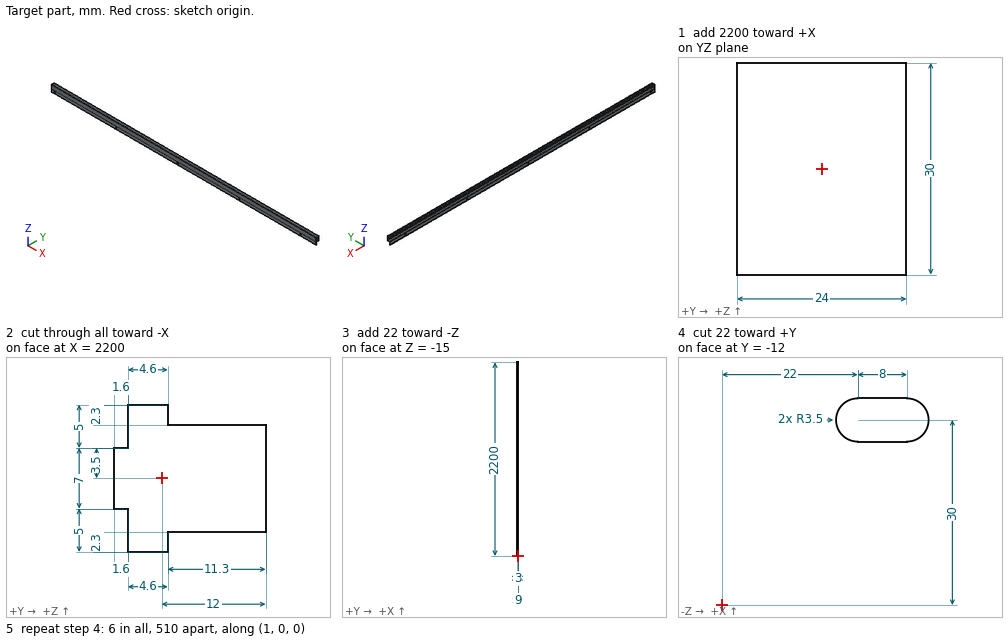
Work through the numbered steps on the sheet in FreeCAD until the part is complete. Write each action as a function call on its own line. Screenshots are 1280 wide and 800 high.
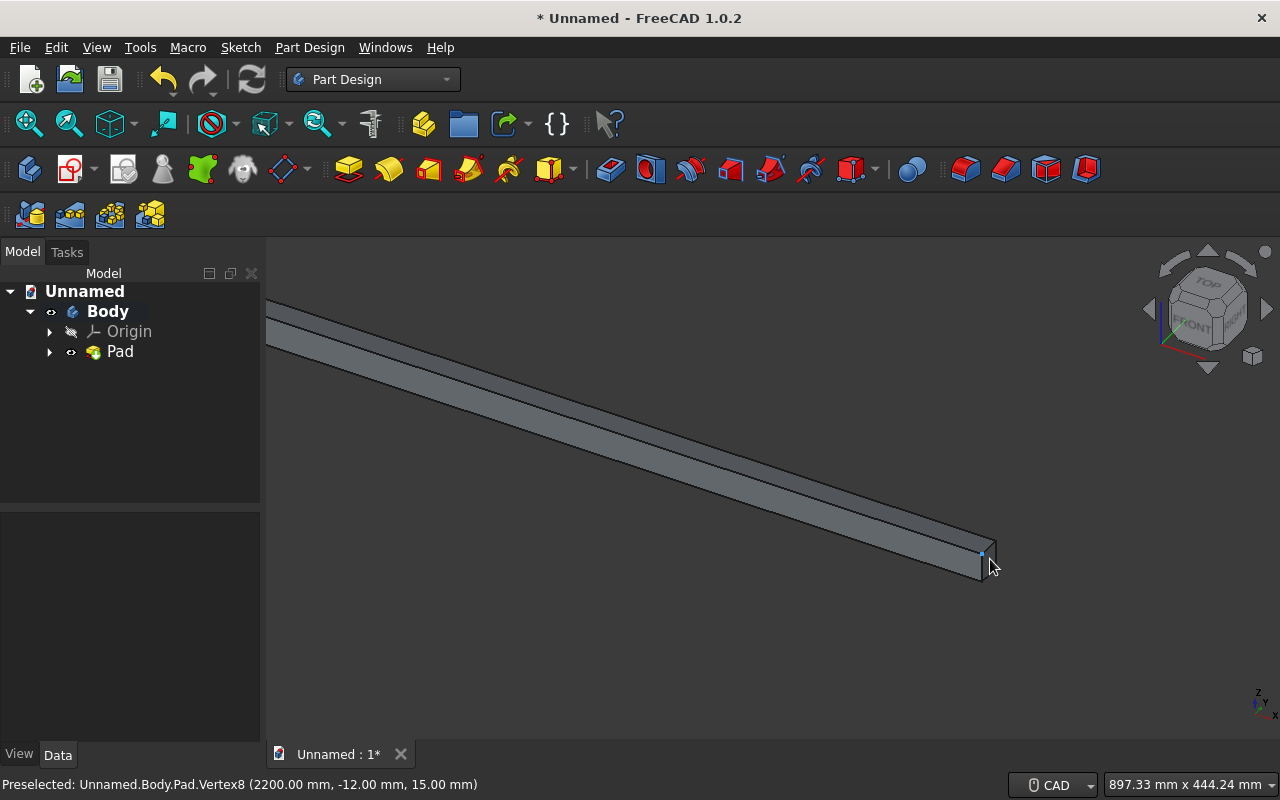
click(991, 562)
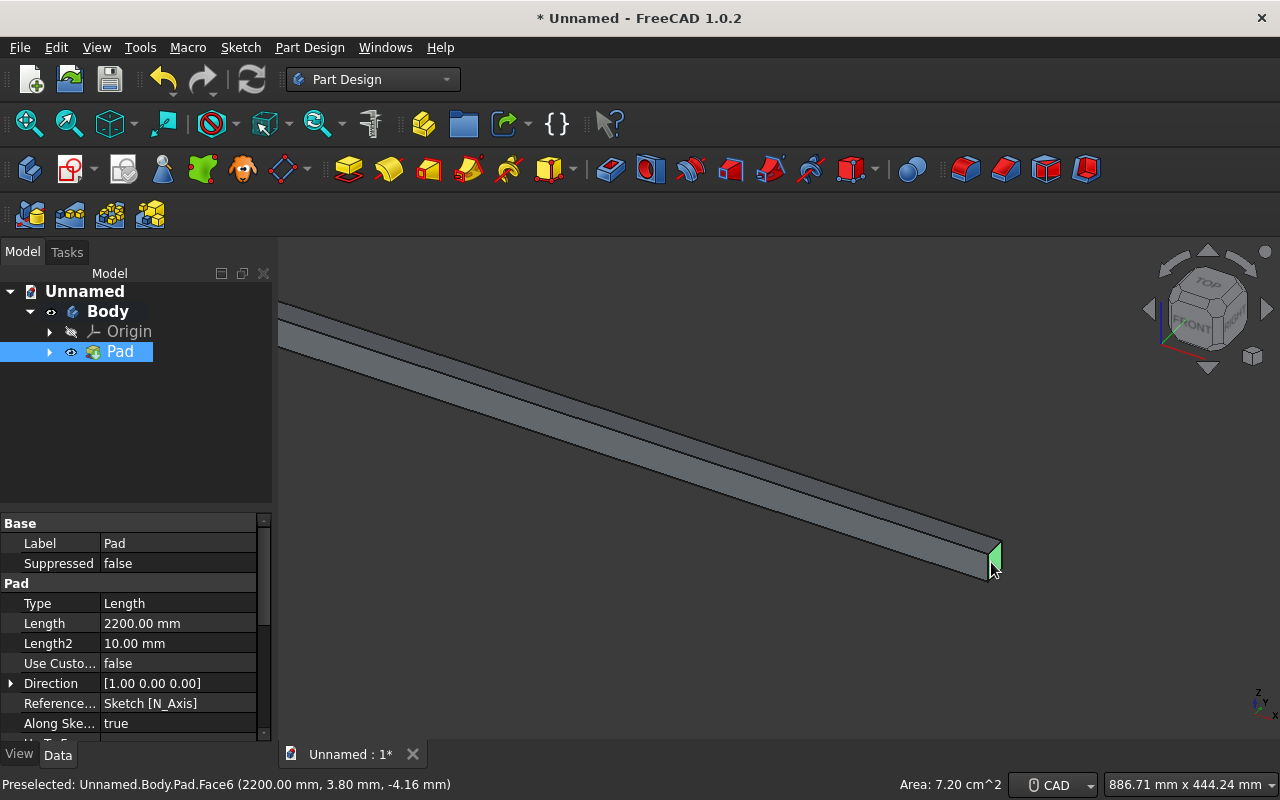
click(70, 170)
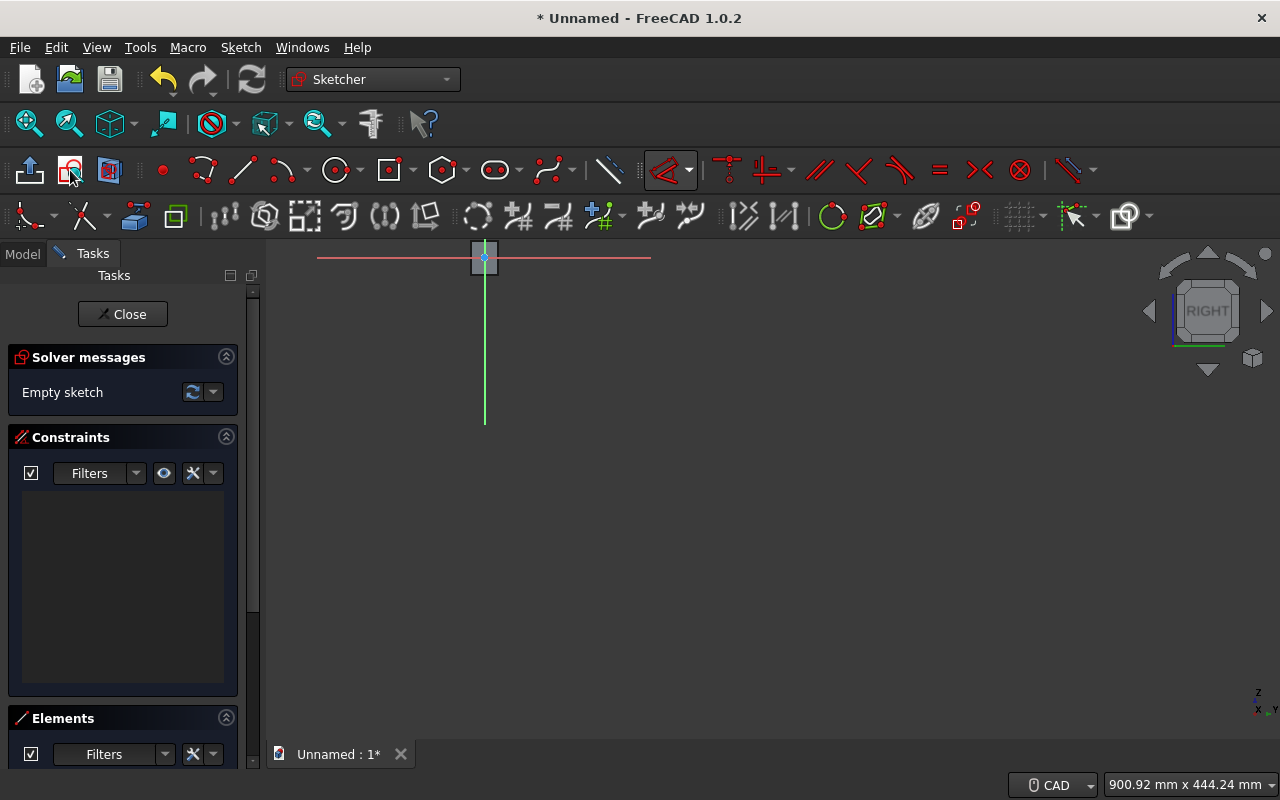
scroll(704, 489, down, 5)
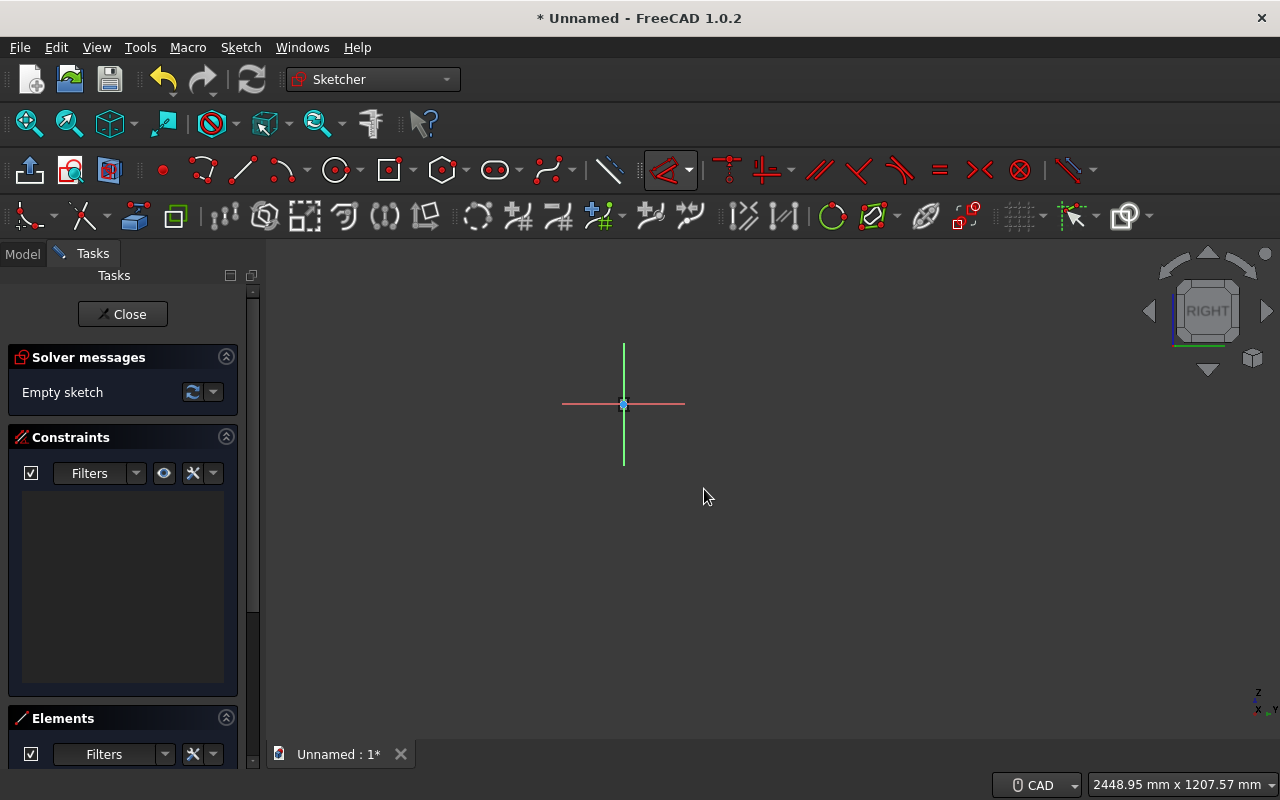
scroll(621, 400, up, 15)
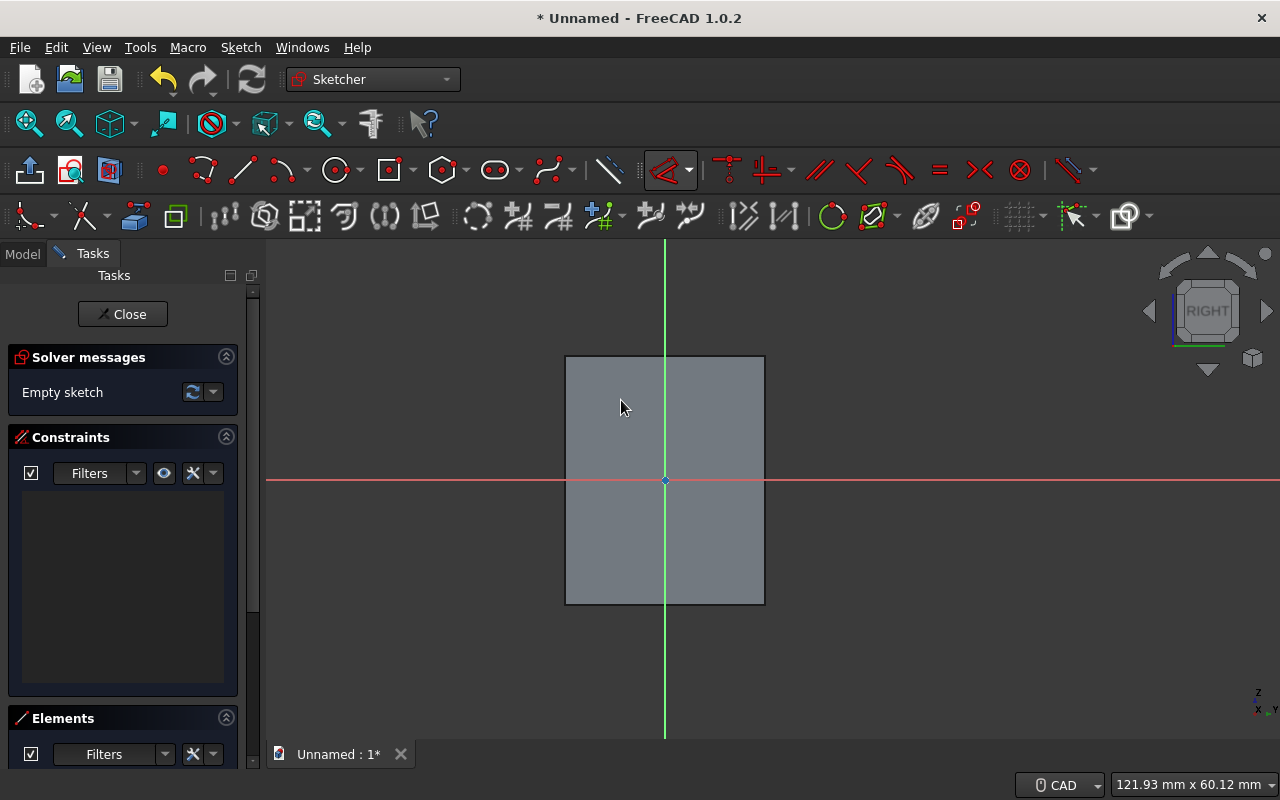
scroll(682, 474, up, 4)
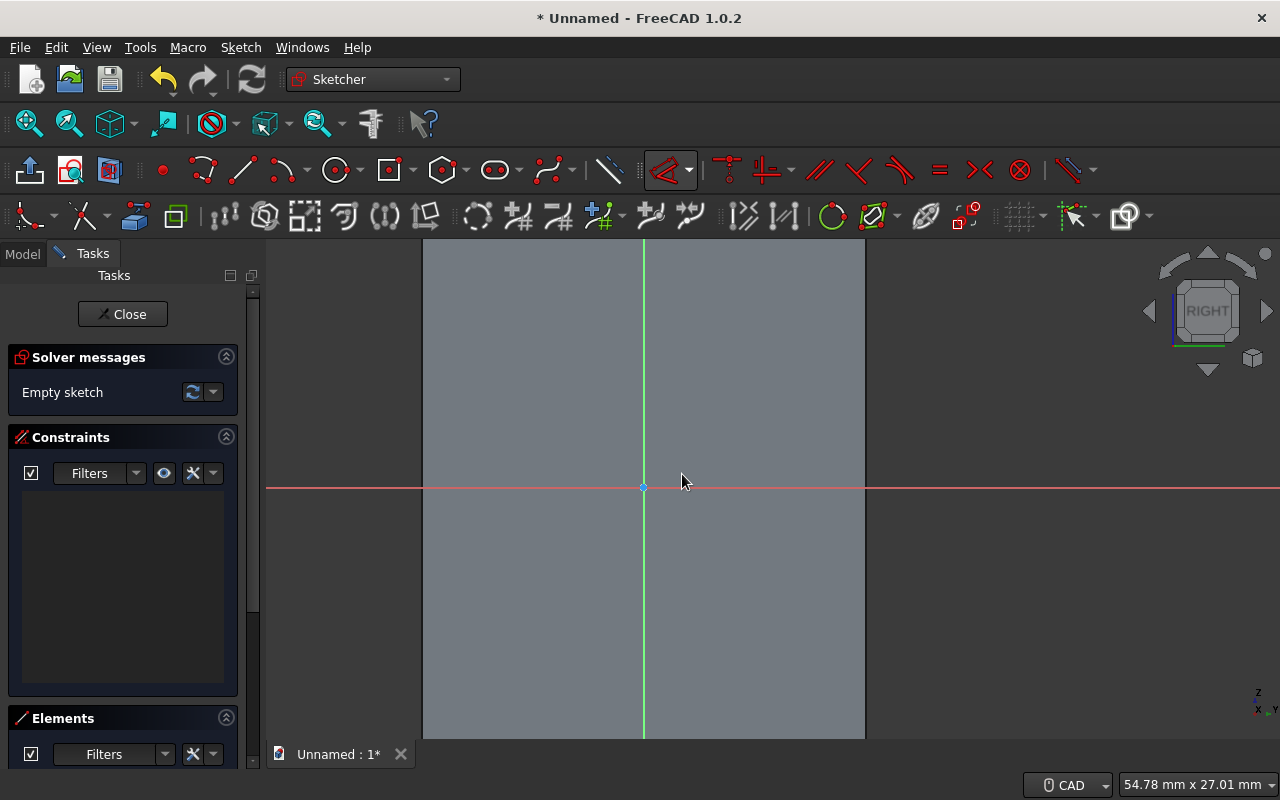
click(204, 170)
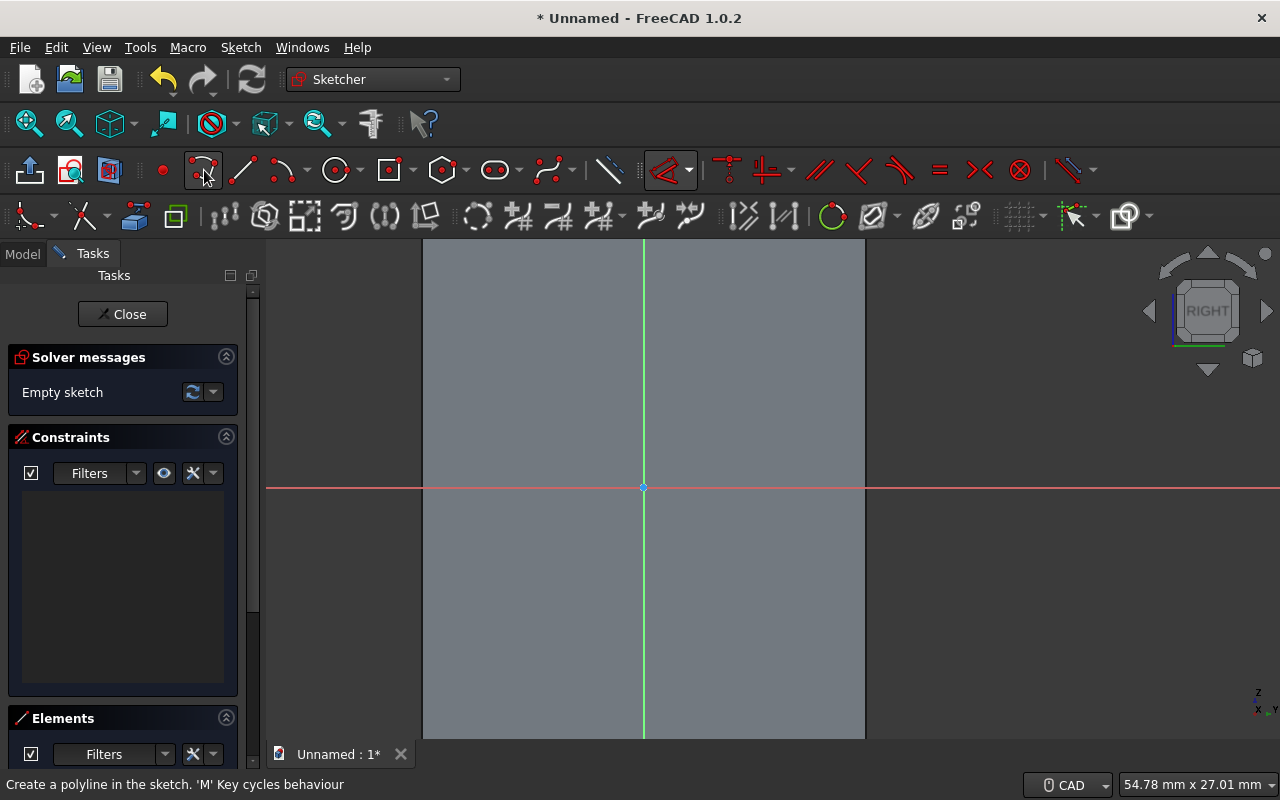
click(572, 423)
click(542, 423)
click(542, 553)
click(572, 553)
click(572, 645)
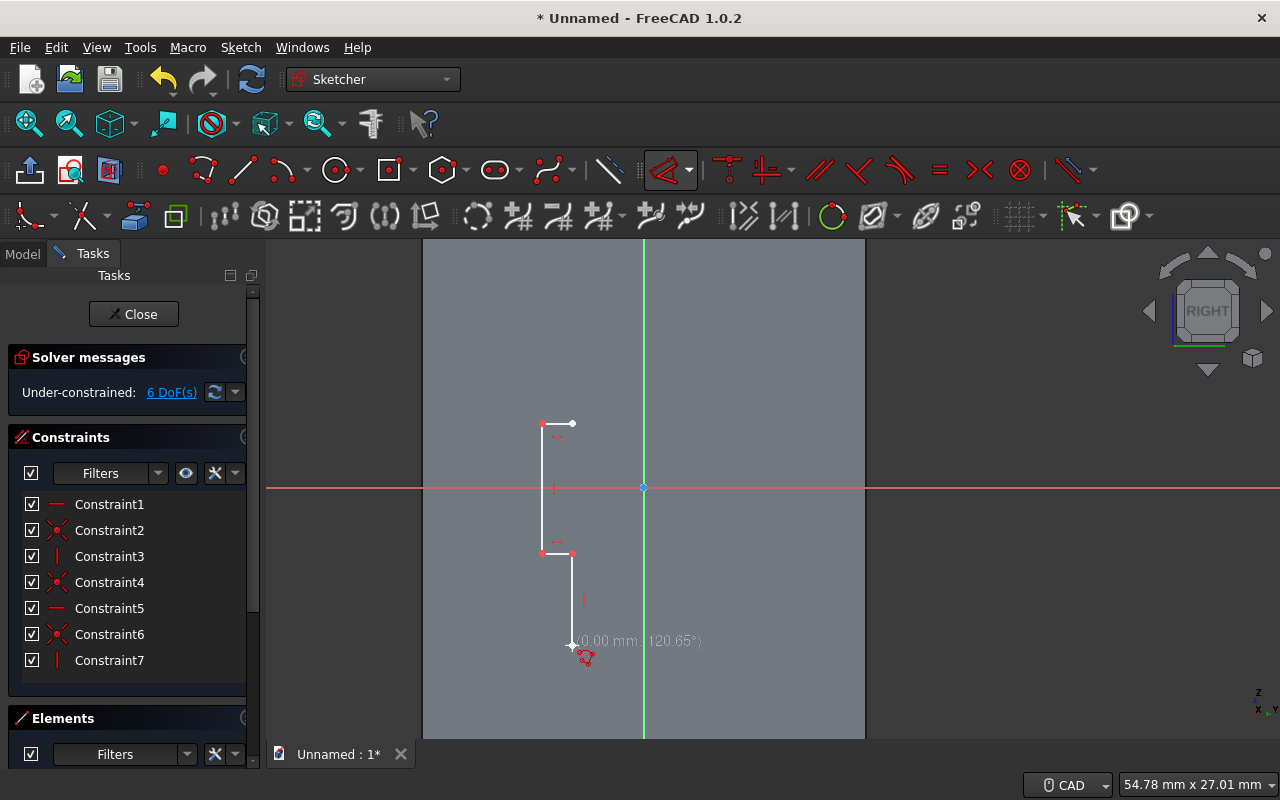
scroll(657, 645, up, 2)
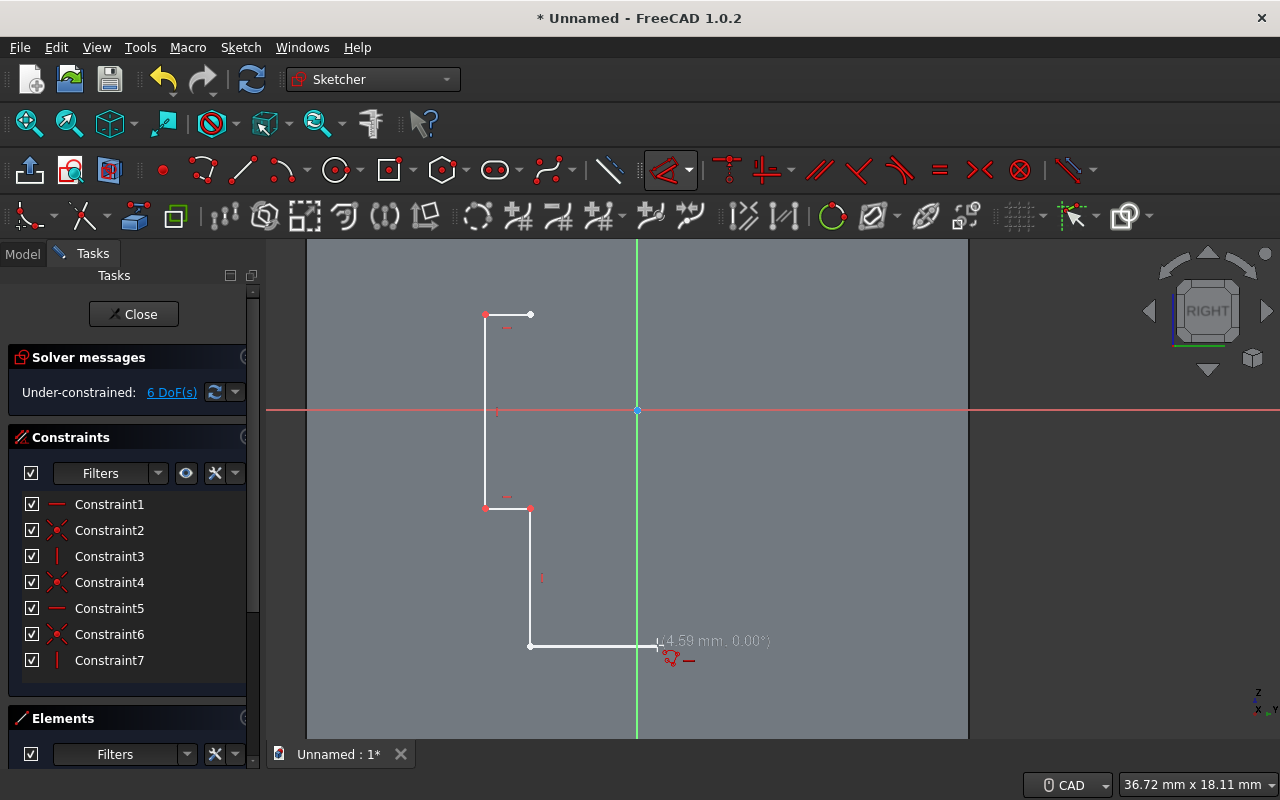
click(657, 645)
click(657, 581)
click(969, 581)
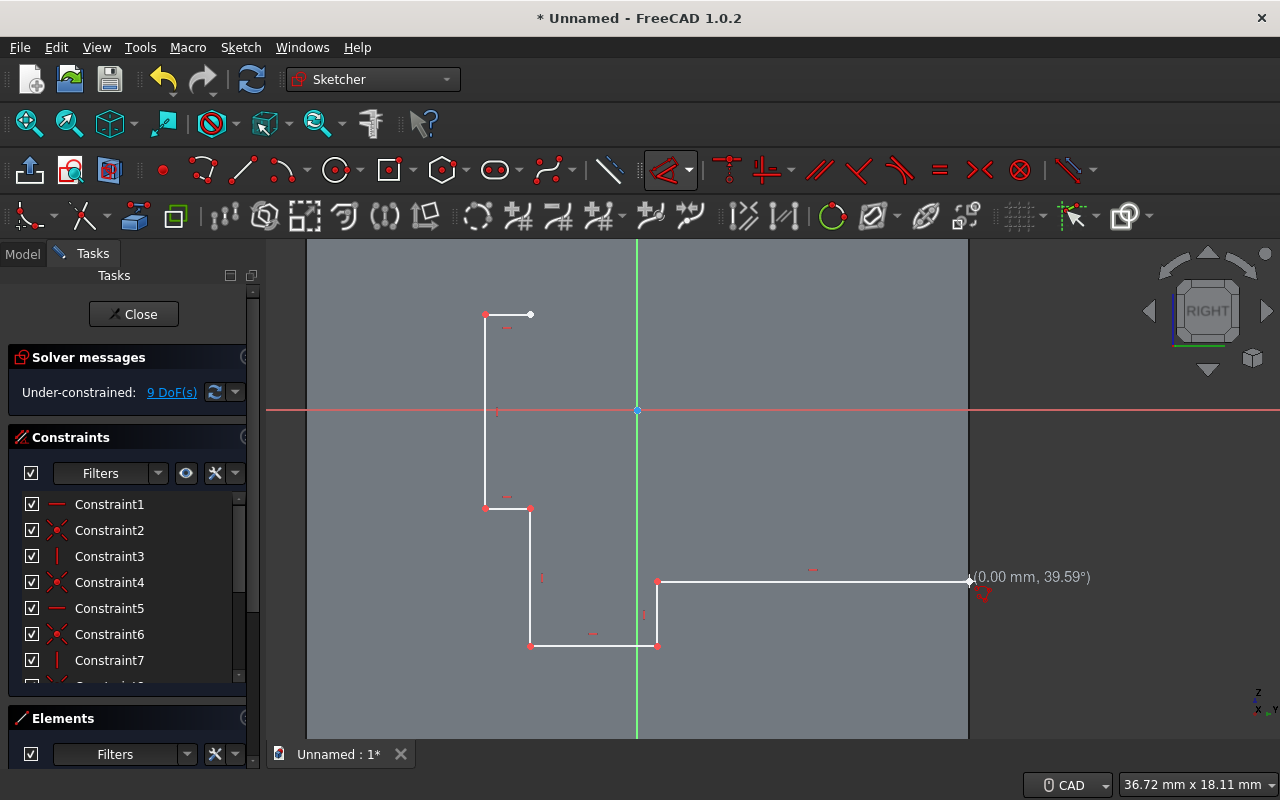
scroll(659, 649, down, 2)